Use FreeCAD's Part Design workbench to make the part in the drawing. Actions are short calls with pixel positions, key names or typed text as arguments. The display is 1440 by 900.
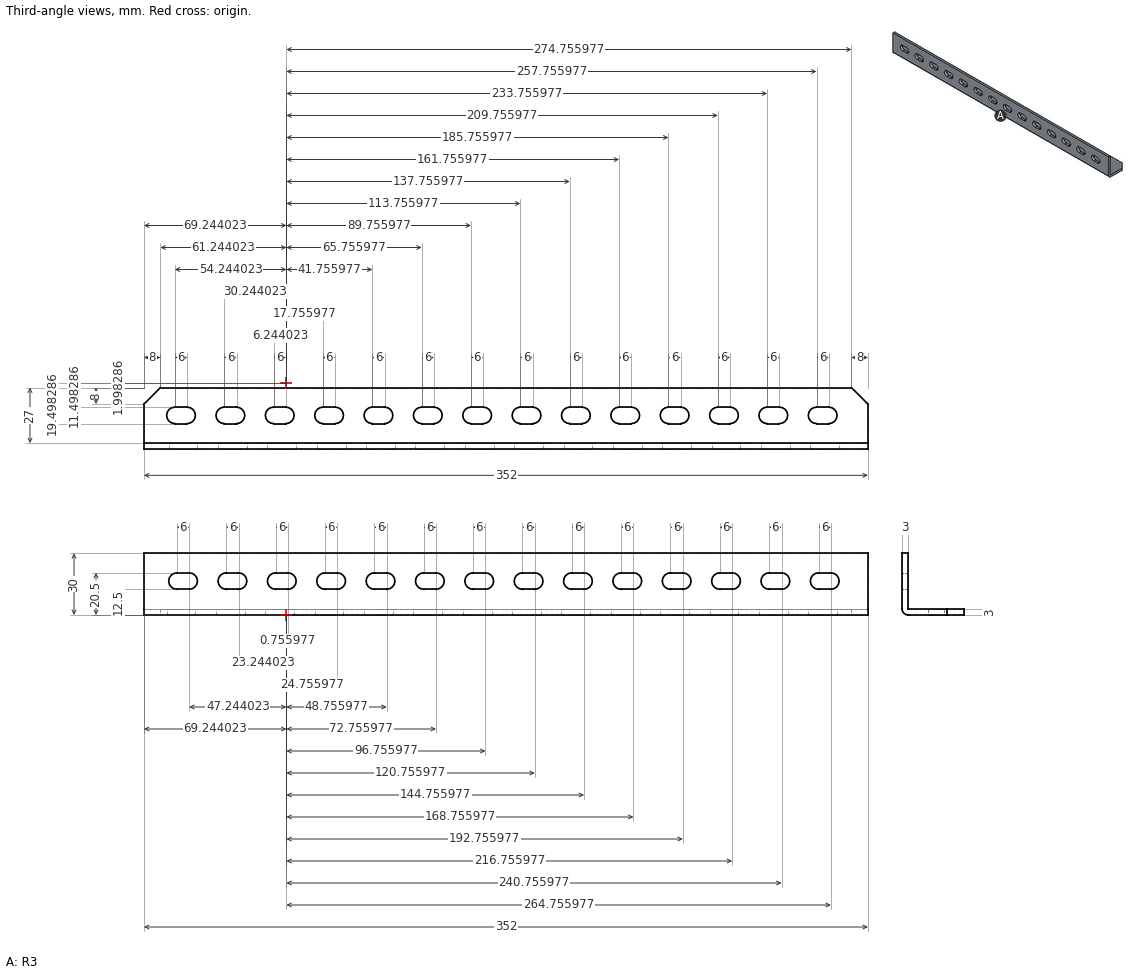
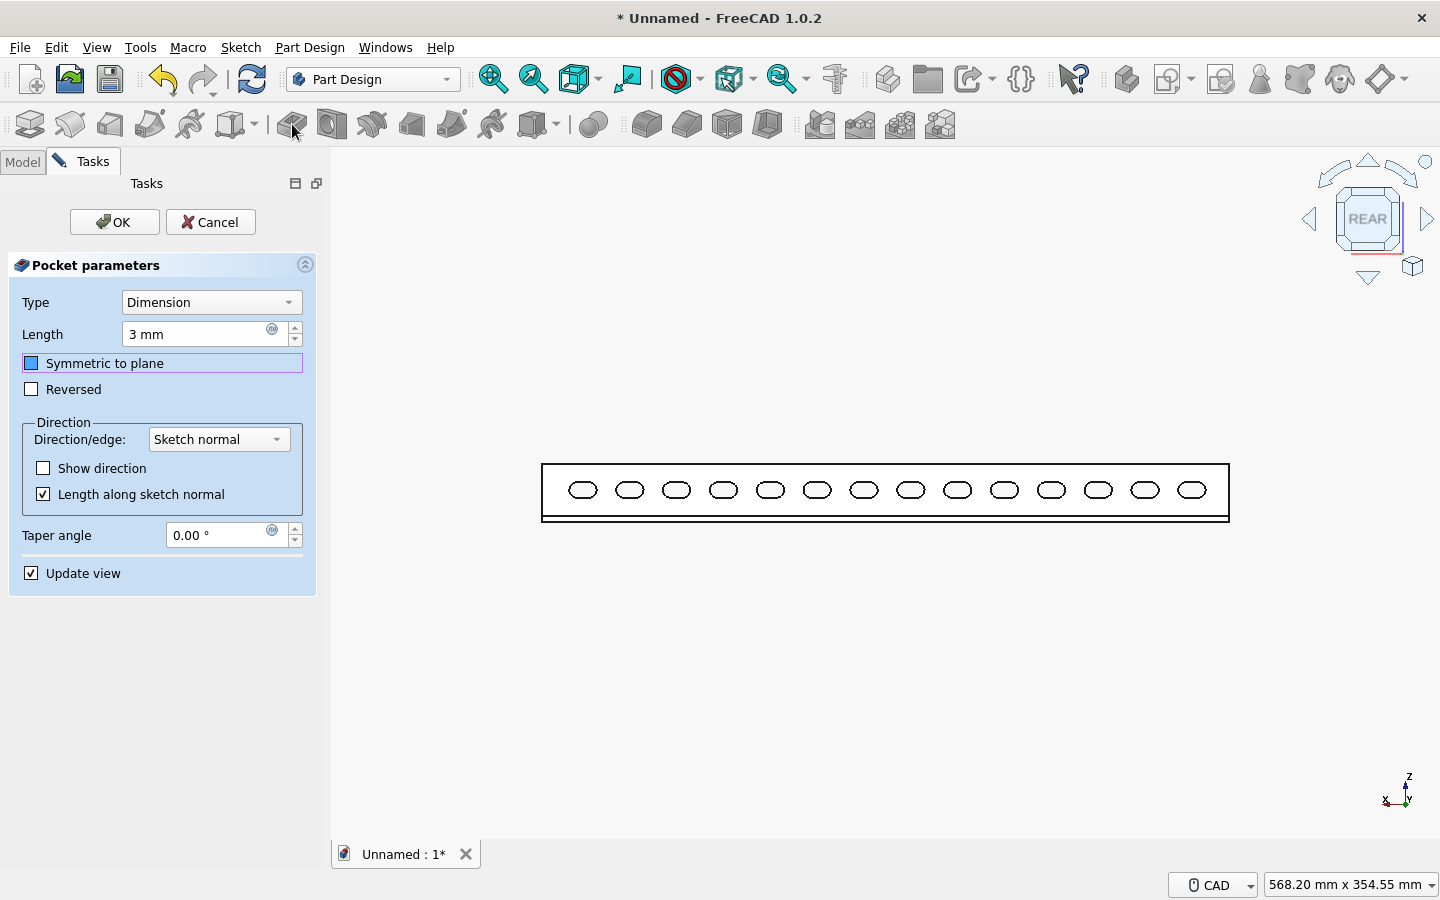
click(115, 222)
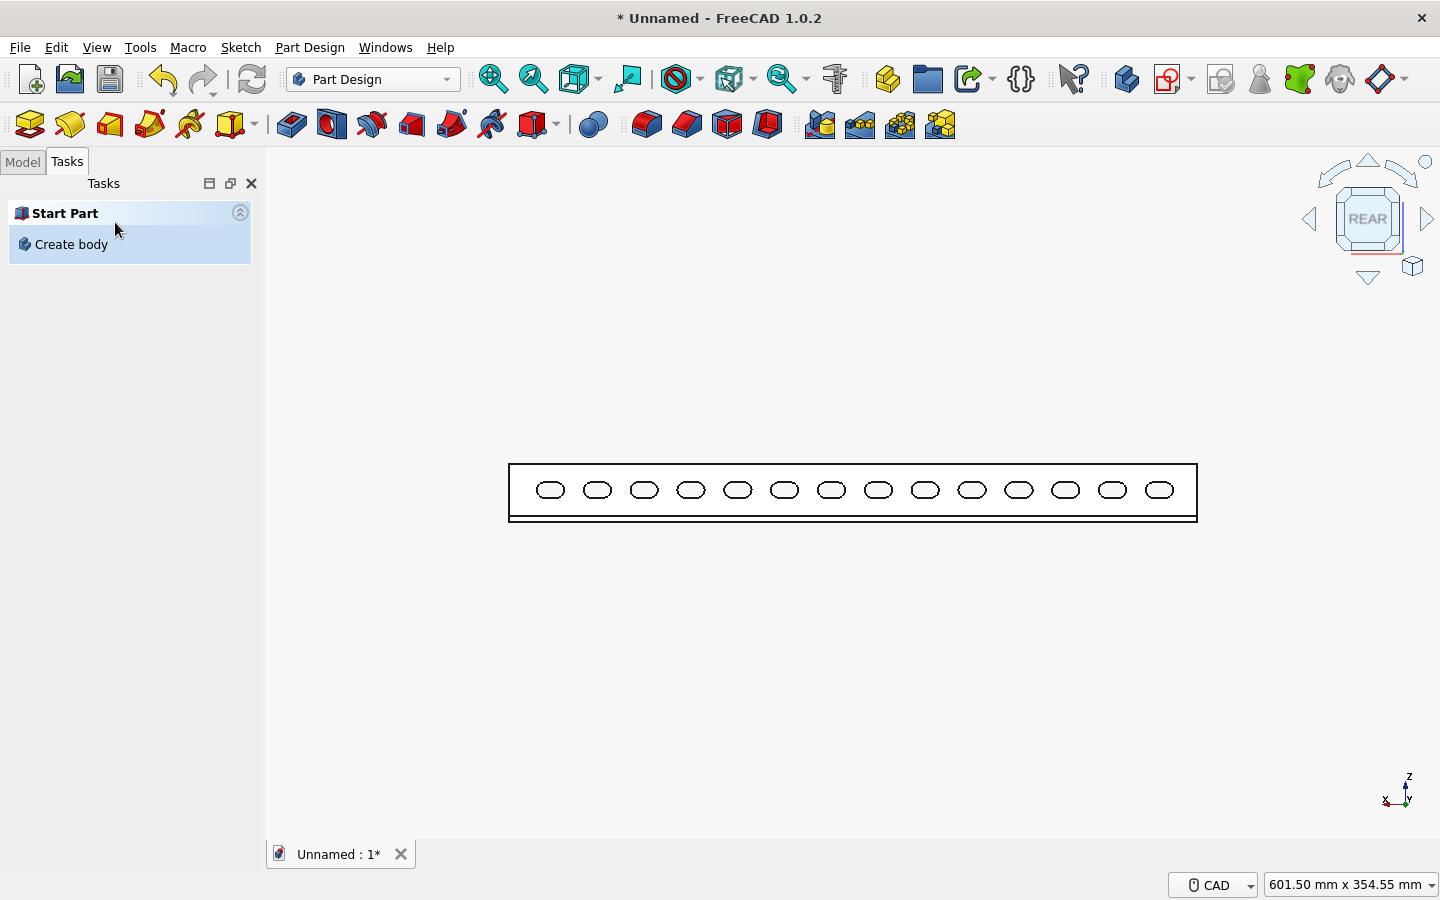
key(0)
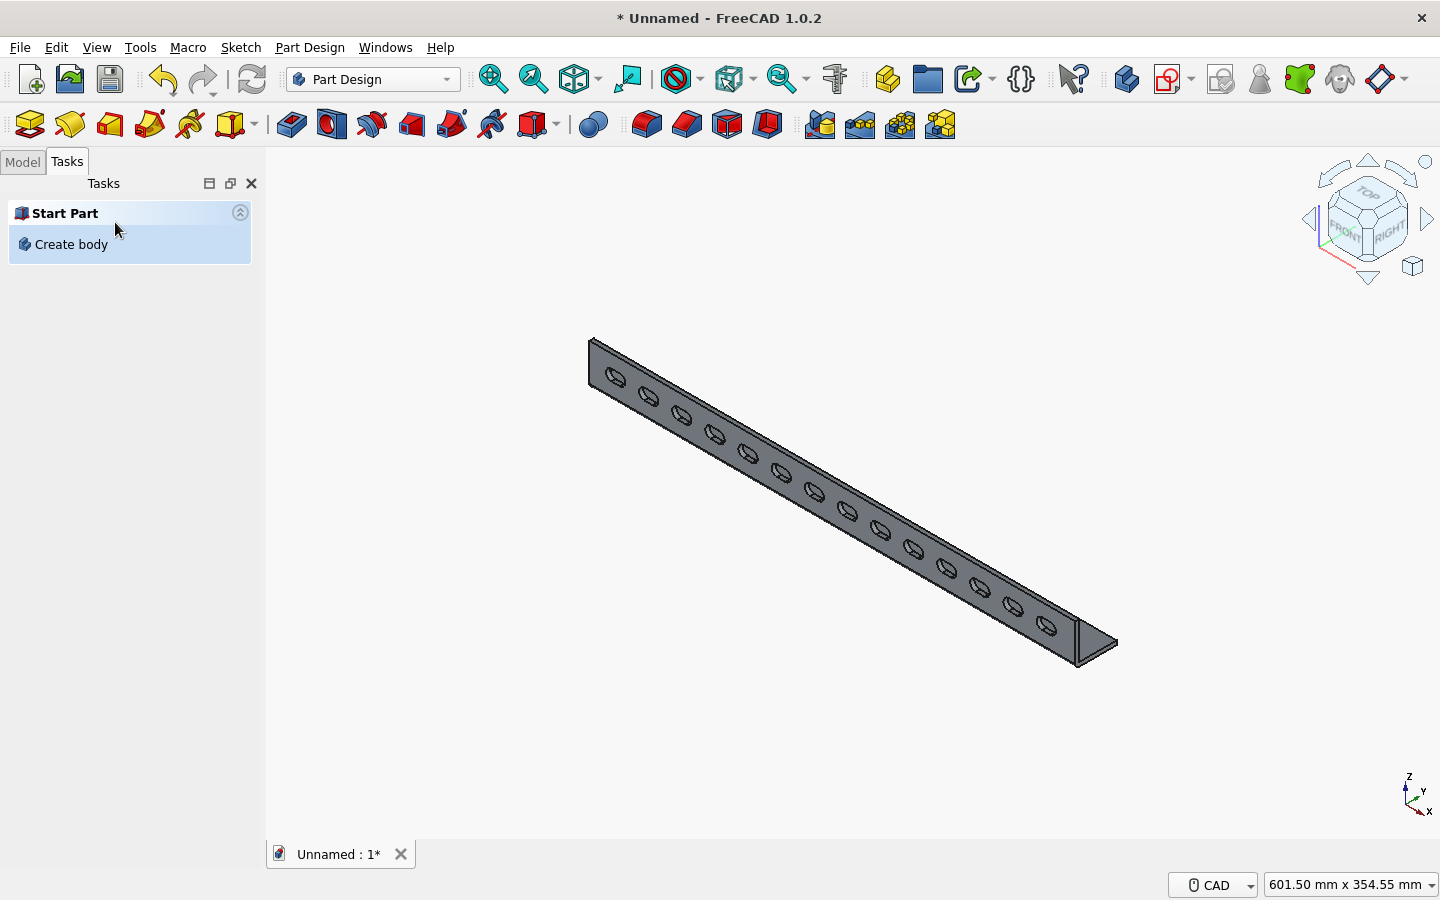
key(2)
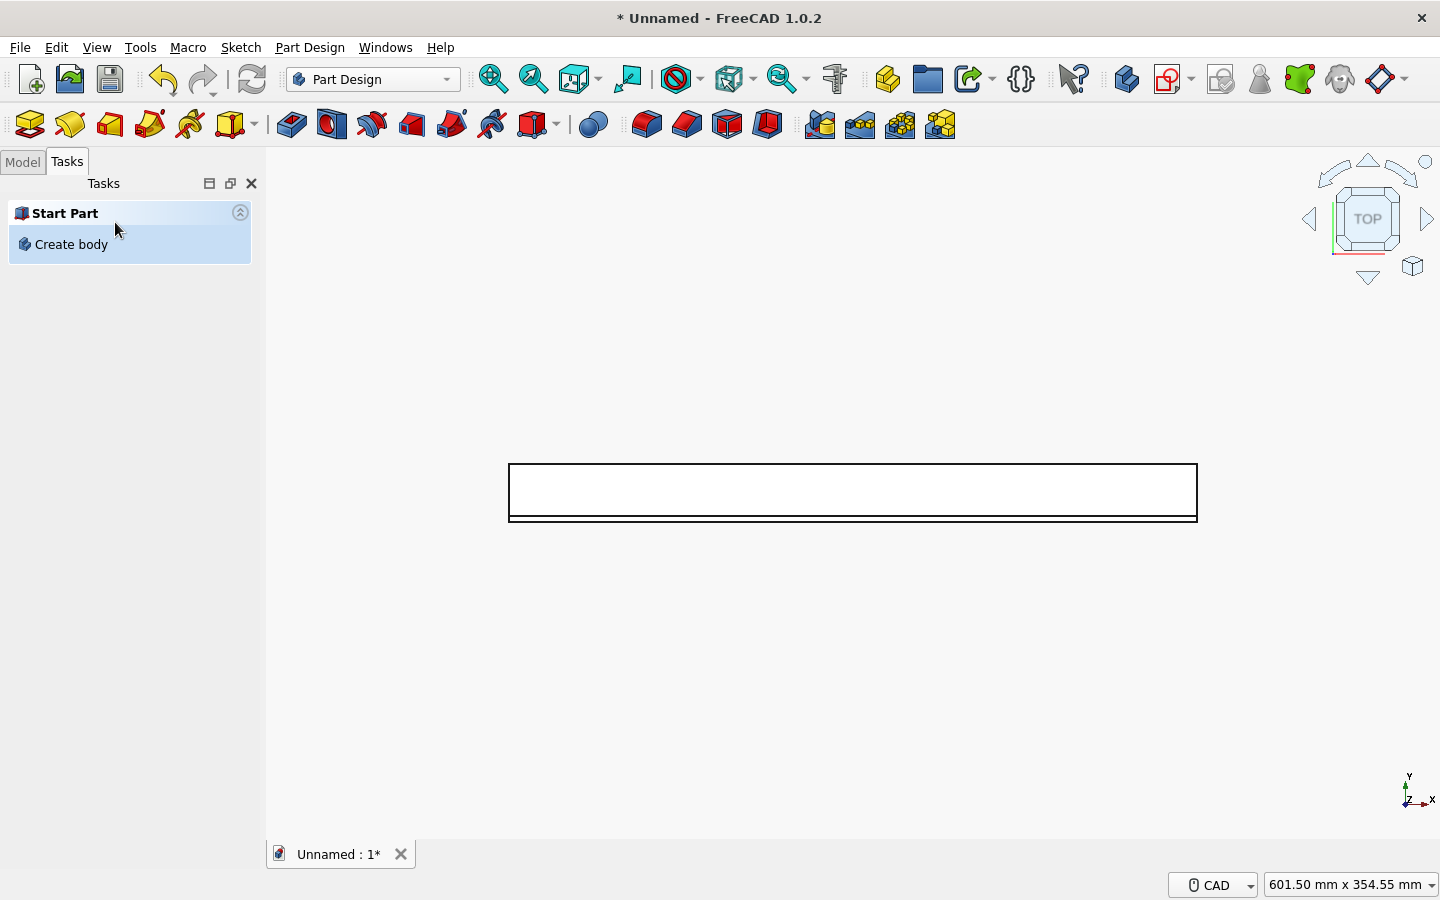
click(1147, 489)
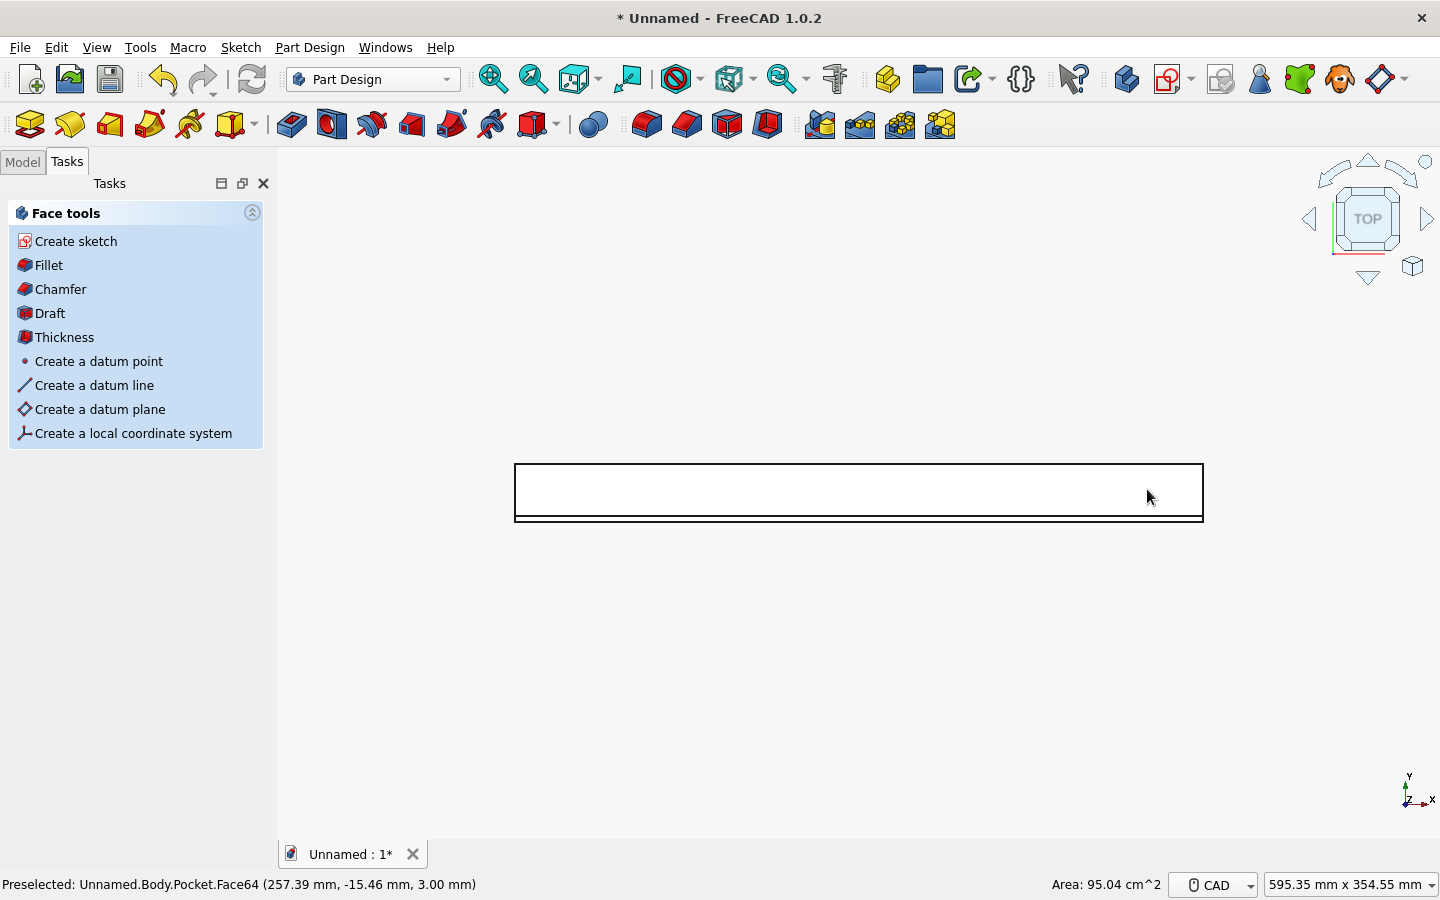
click(1168, 80)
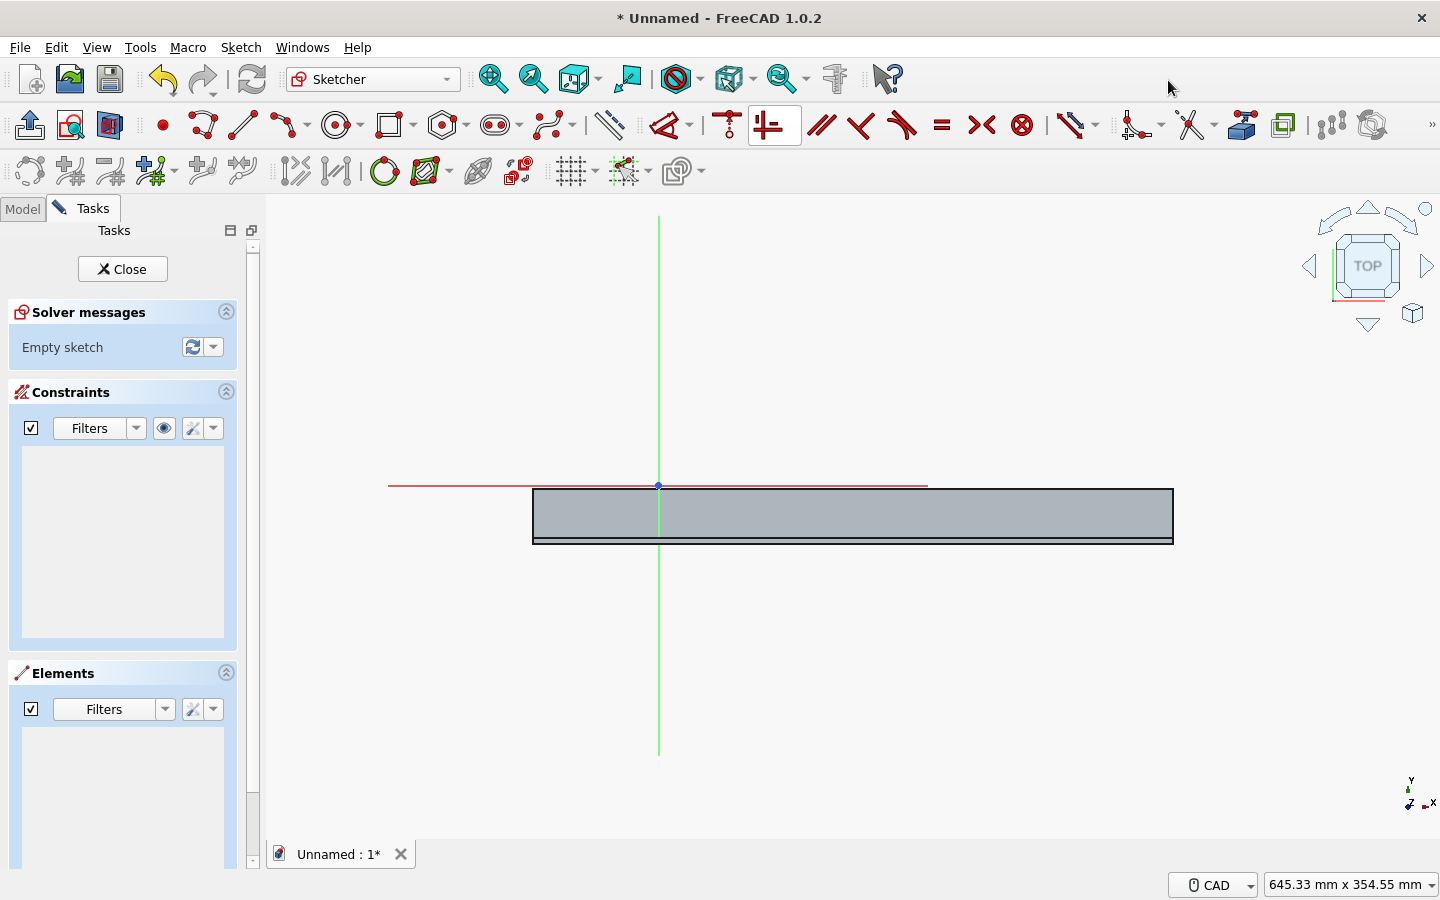
click(110, 126)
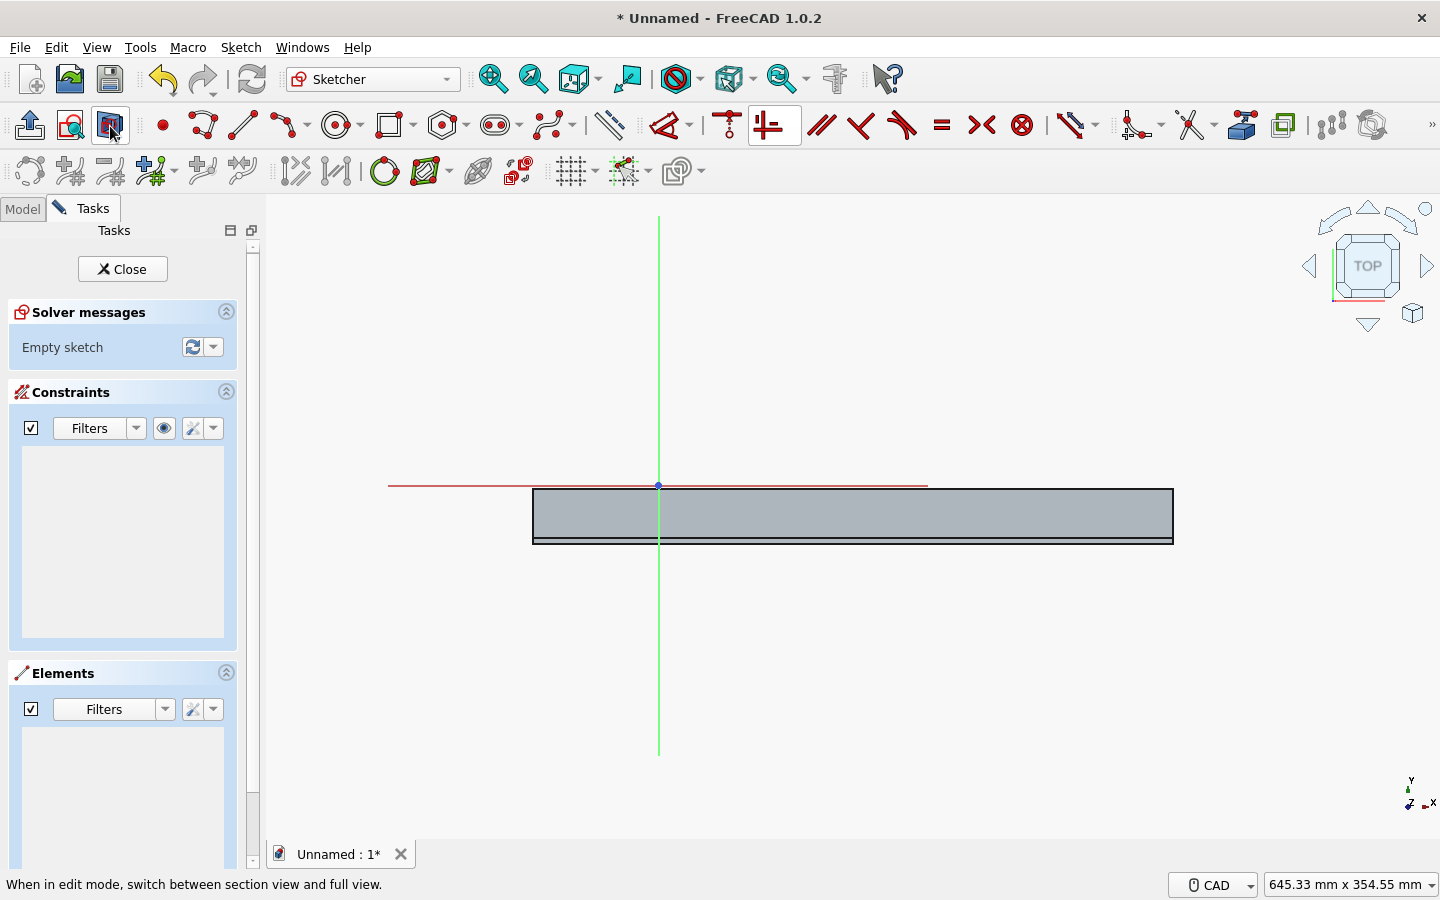
click(496, 126)